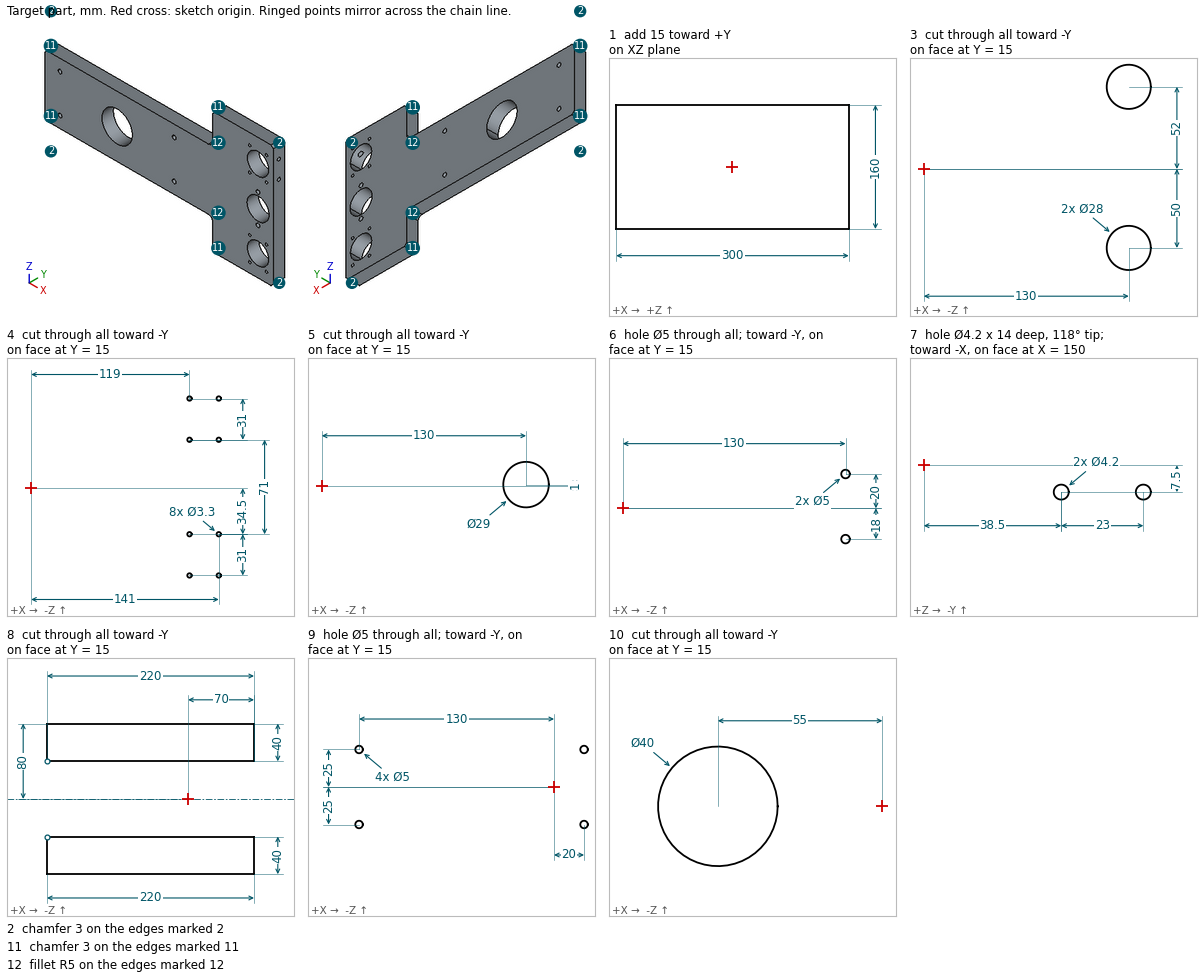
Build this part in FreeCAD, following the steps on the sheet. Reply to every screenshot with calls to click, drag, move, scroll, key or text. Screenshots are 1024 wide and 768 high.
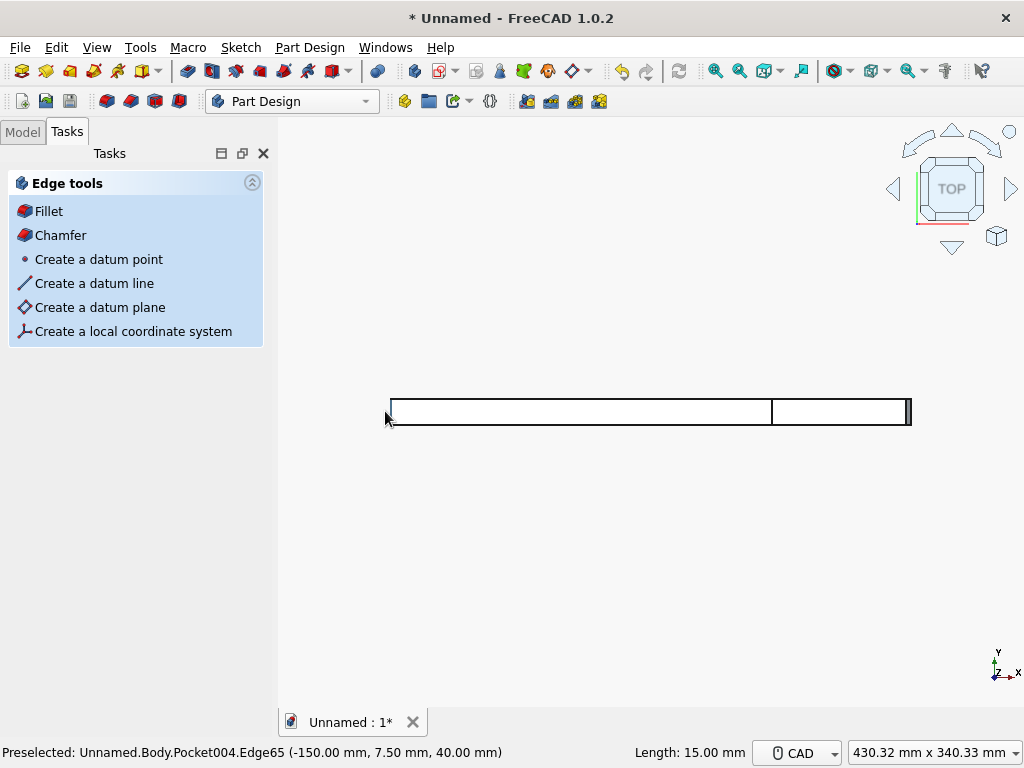
click(772, 411, ctrl)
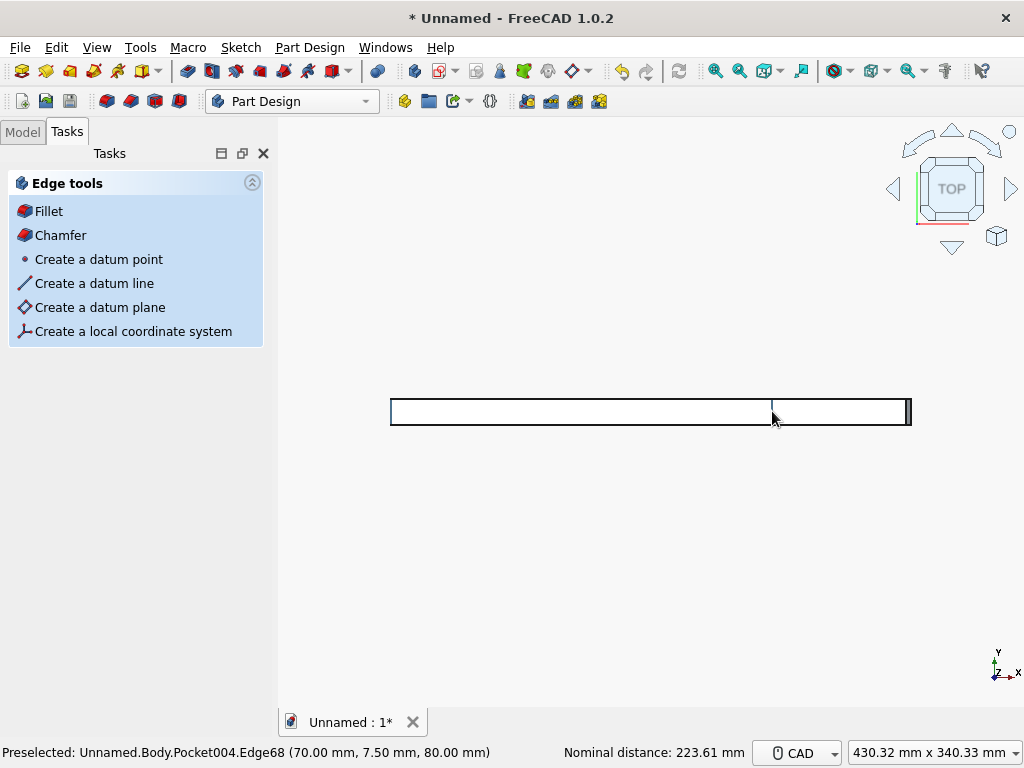
key(1)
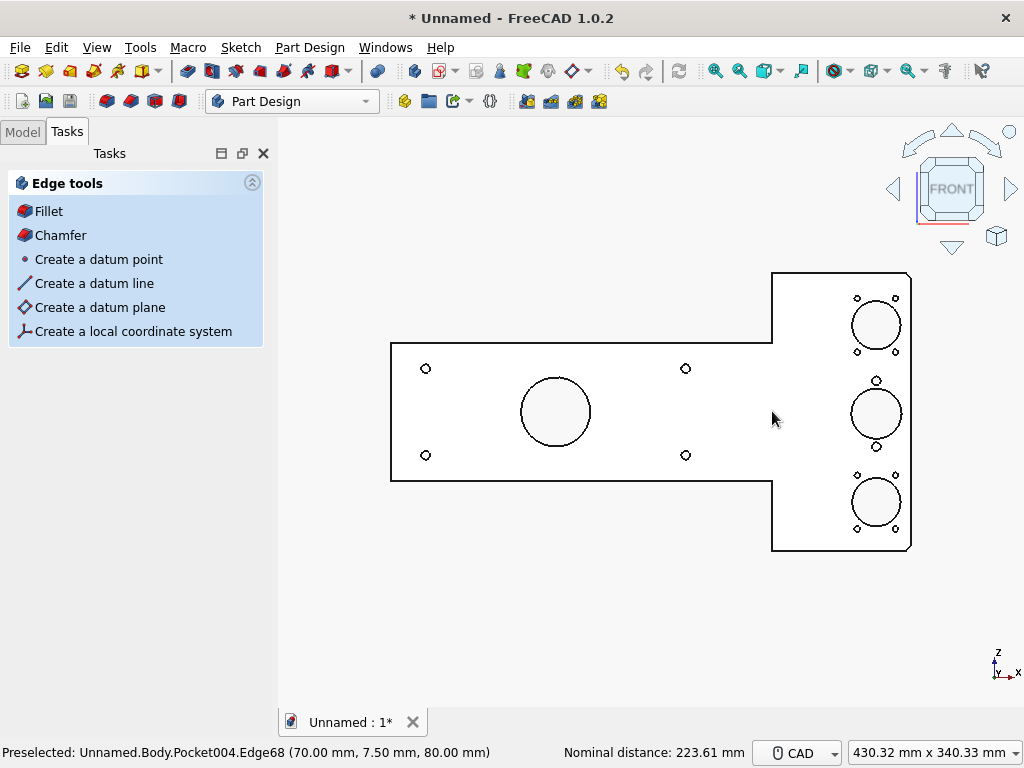
key(3)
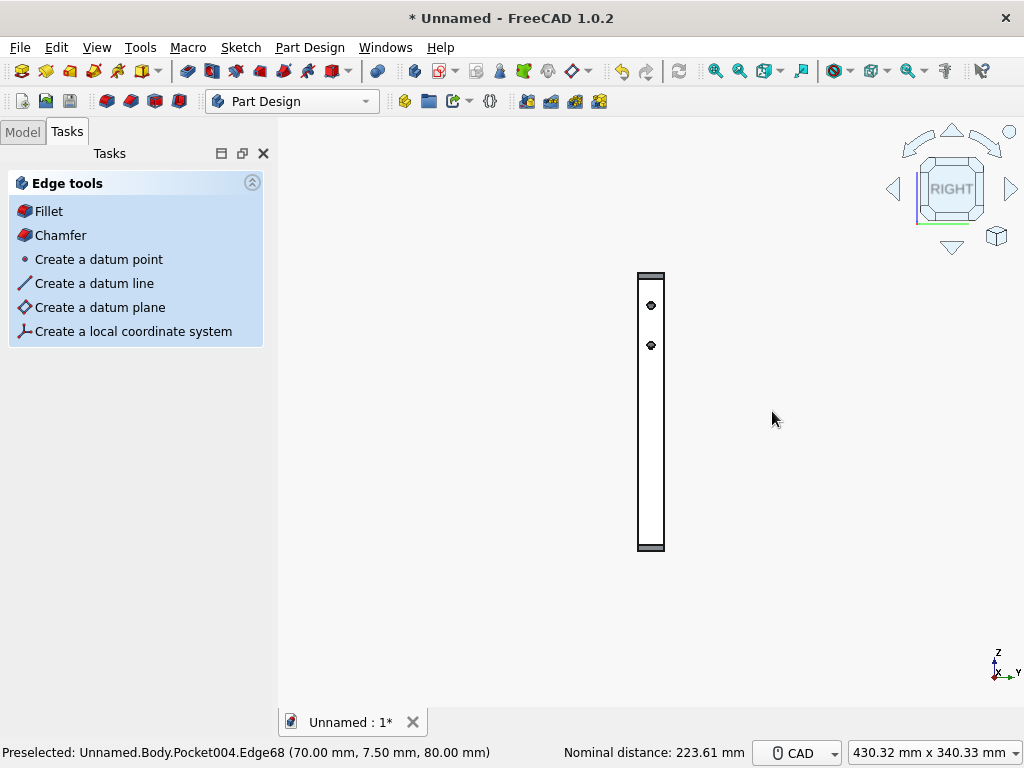
key(5)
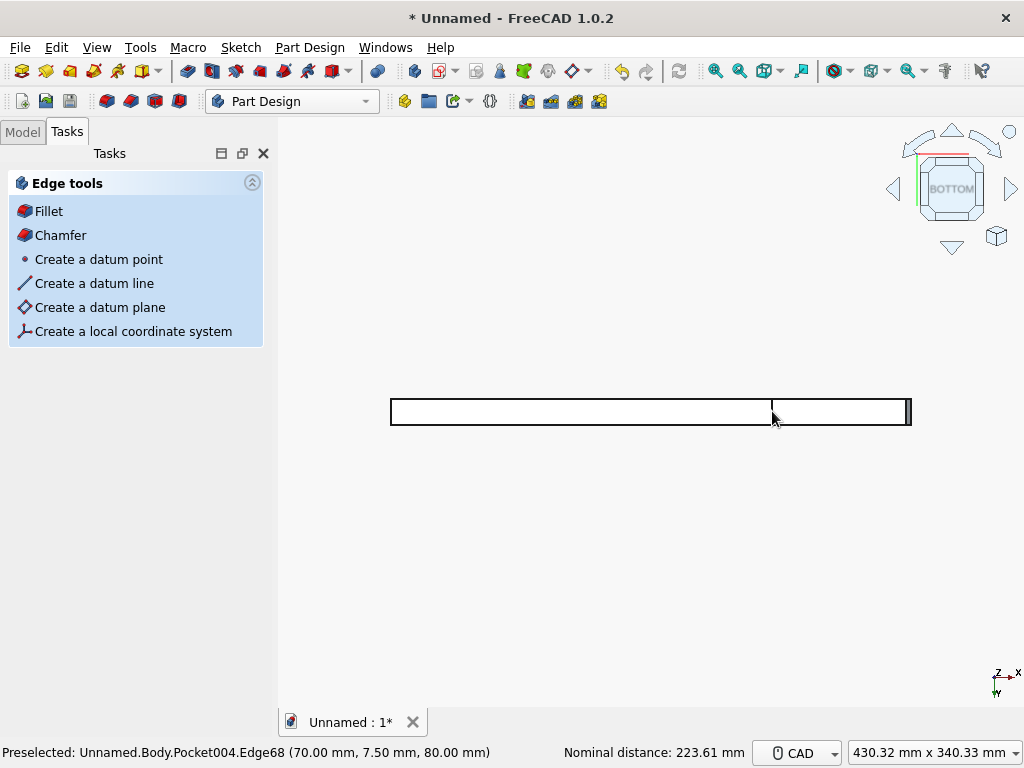
click(772, 411, ctrl)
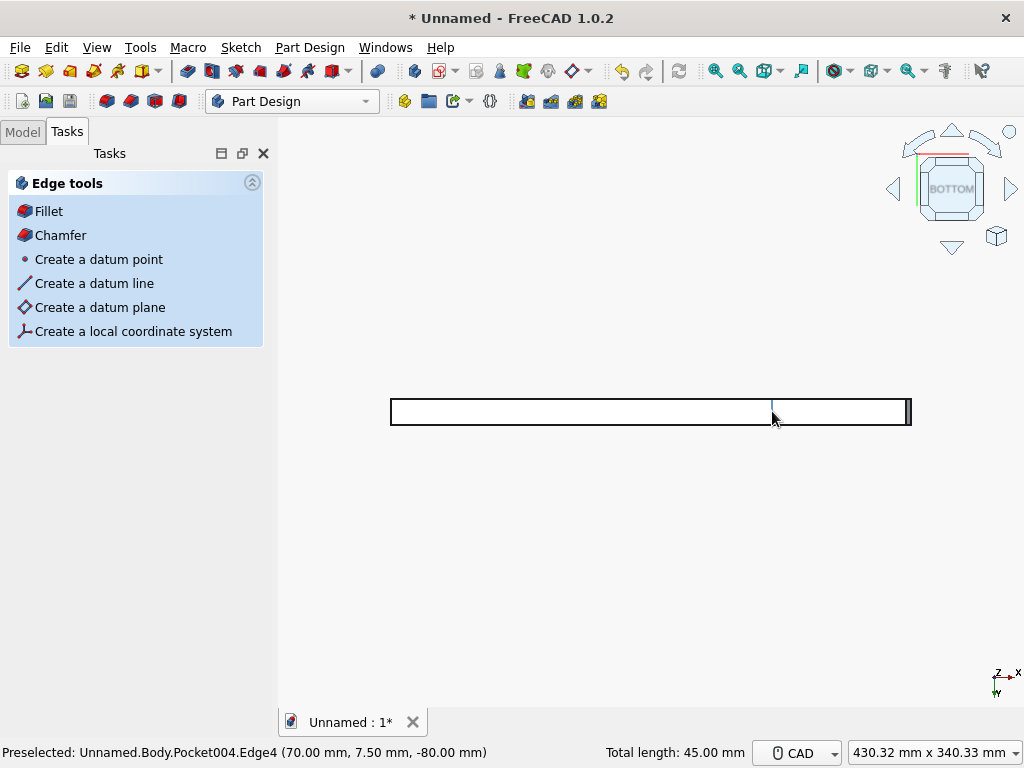
click(391, 411, ctrl)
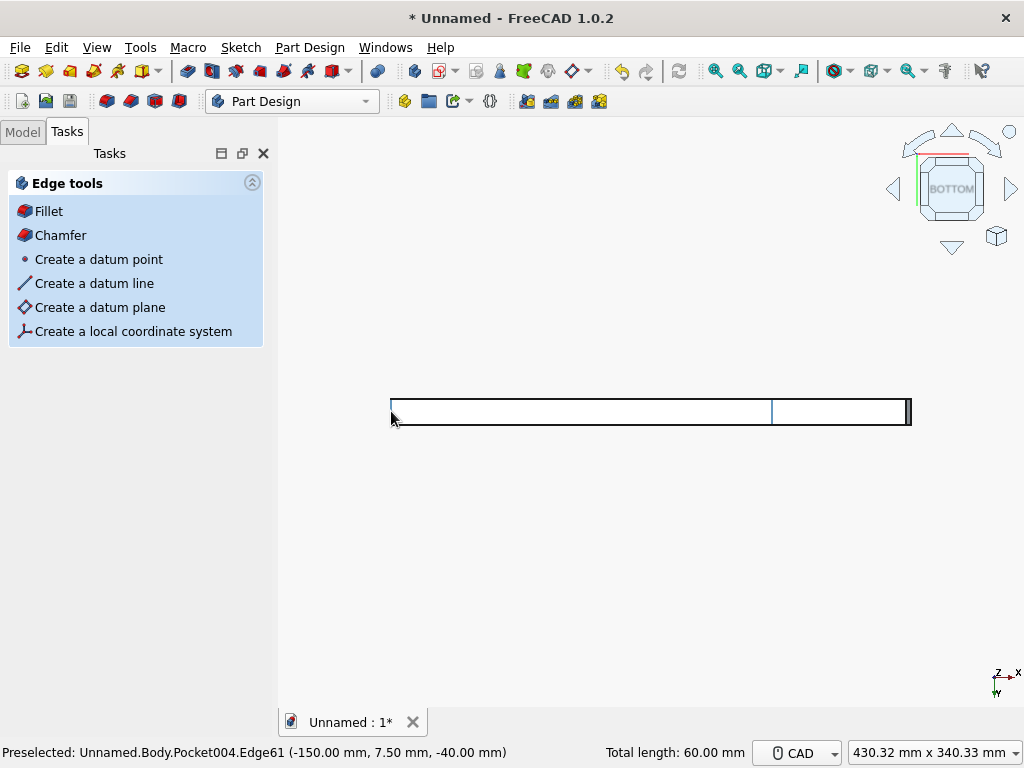
click(132, 102)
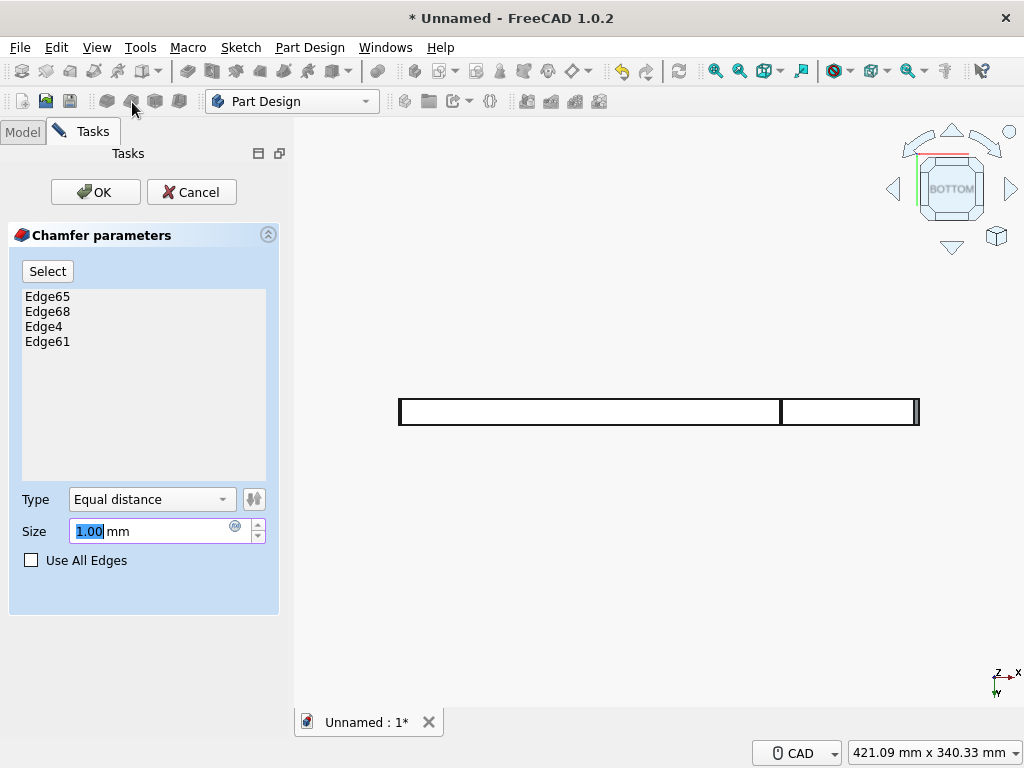
text(3)
key(Tab)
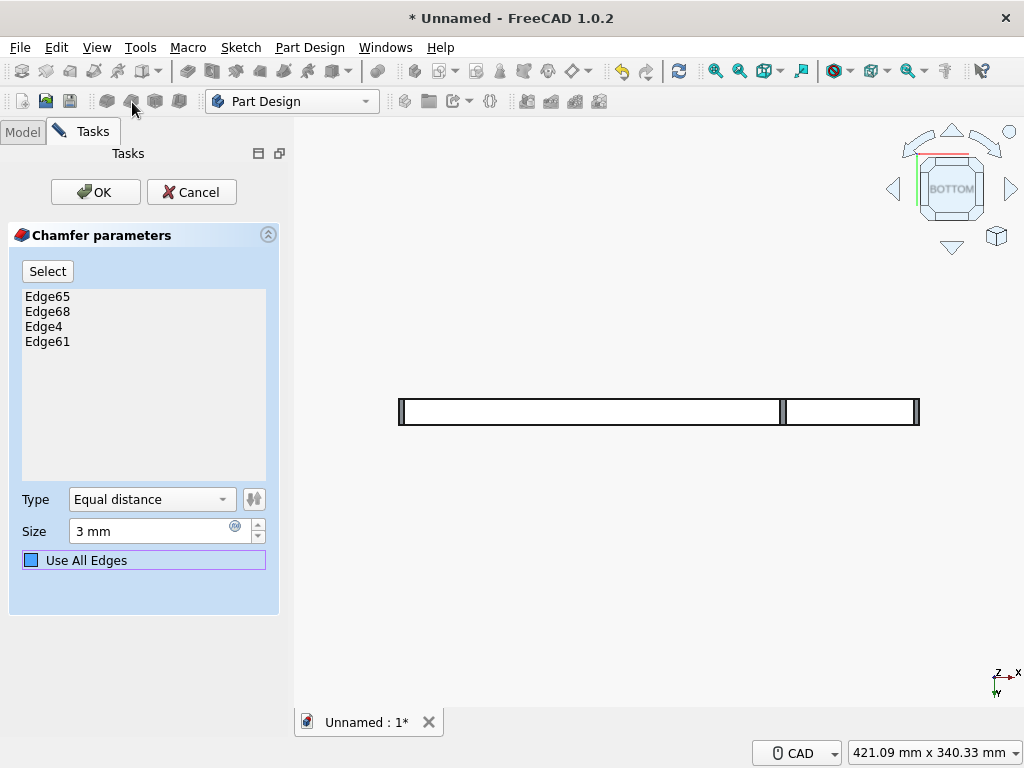
click(96, 192)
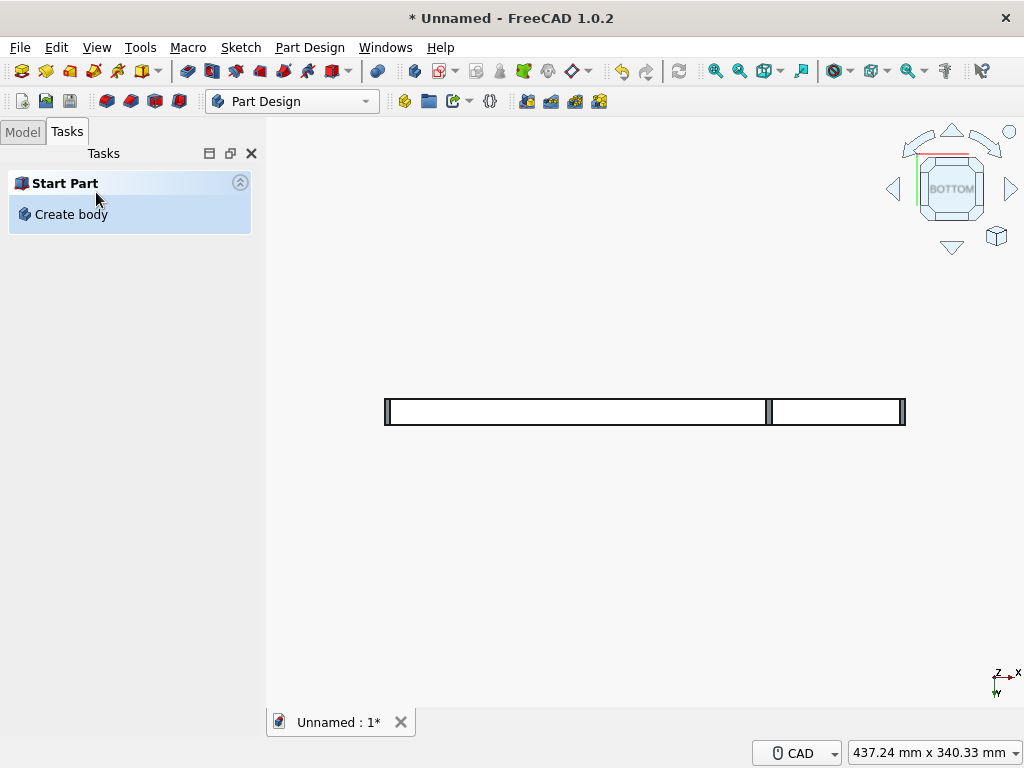
key(0)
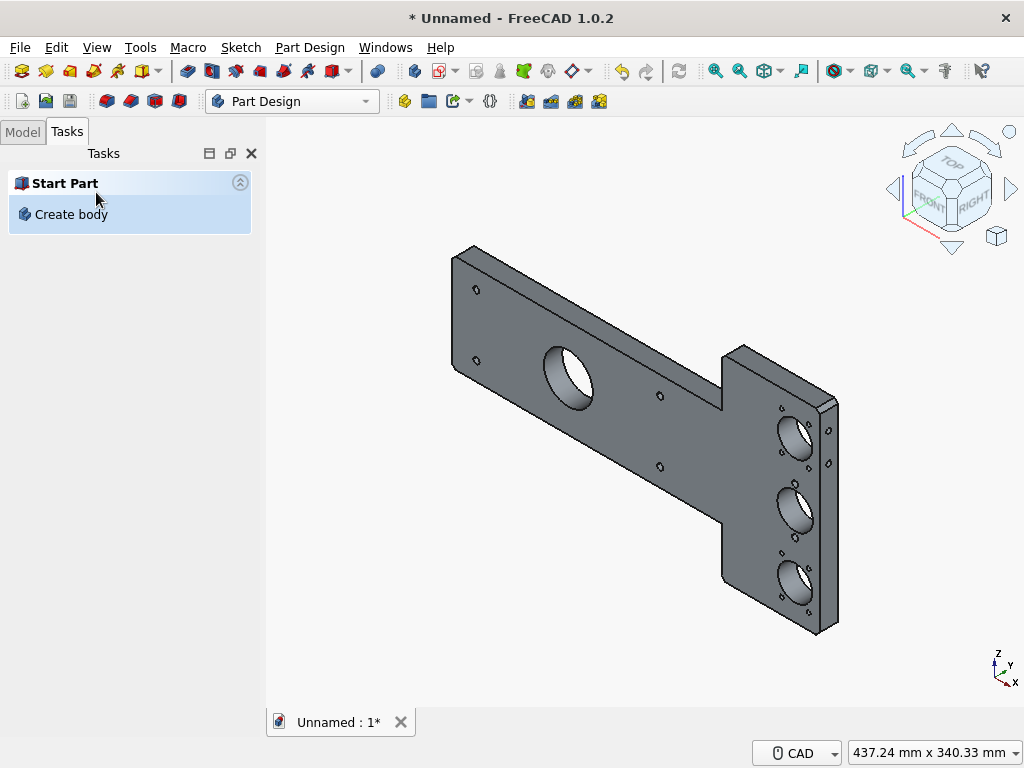
key(2)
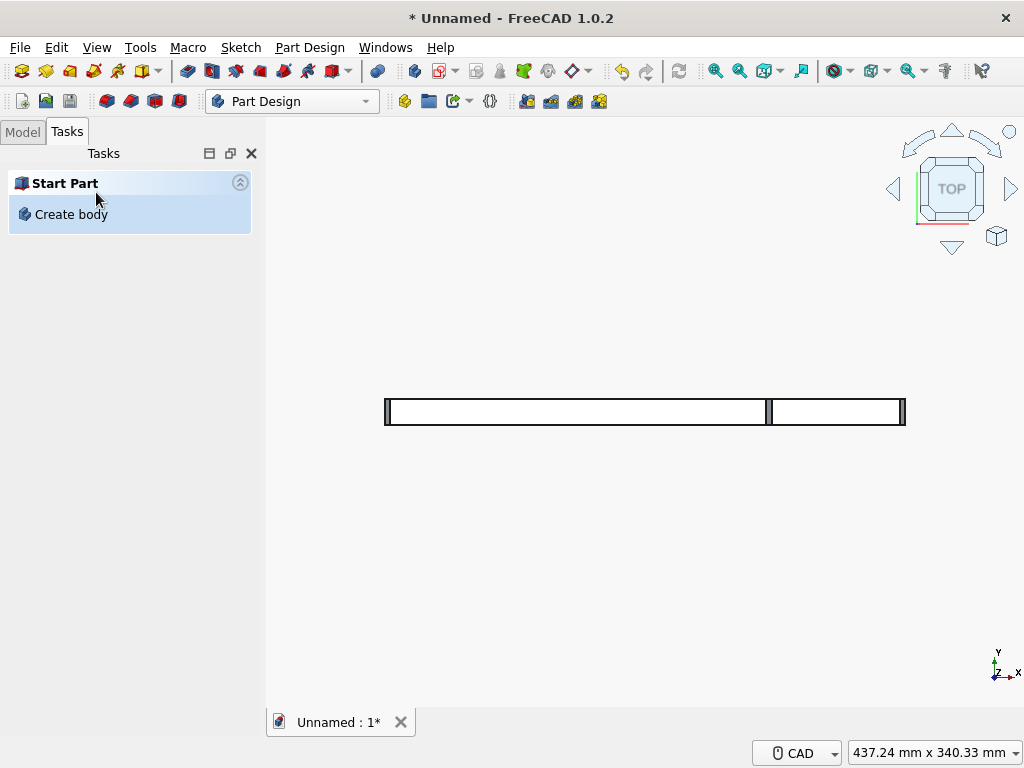
key(1)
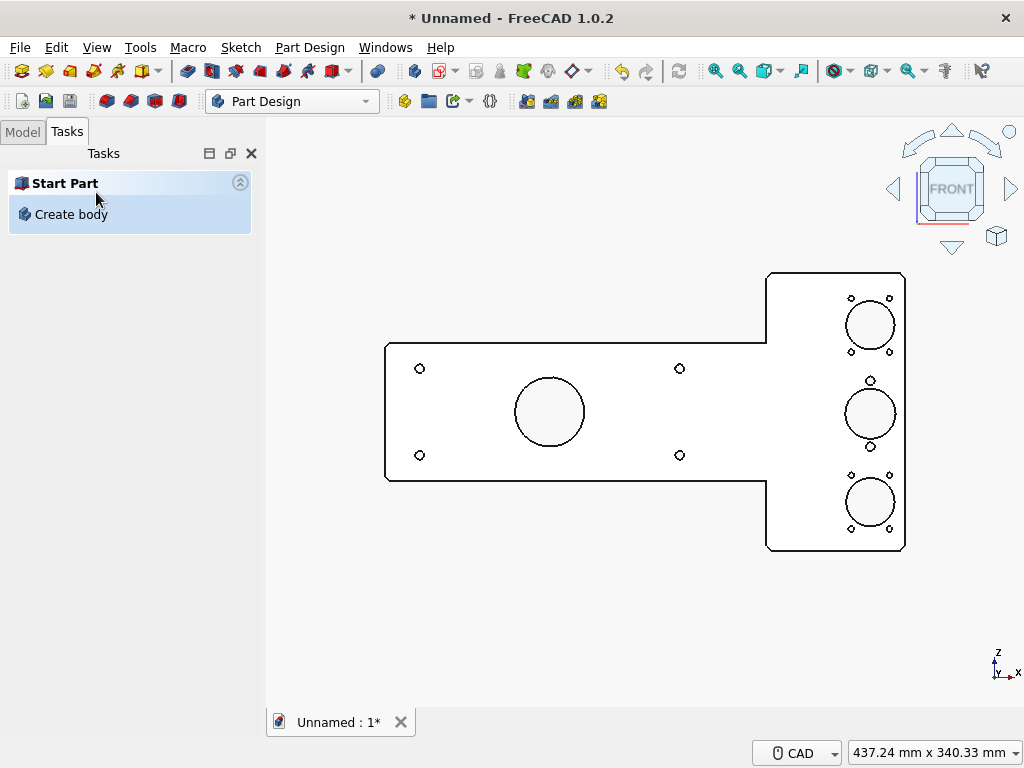
key(3)